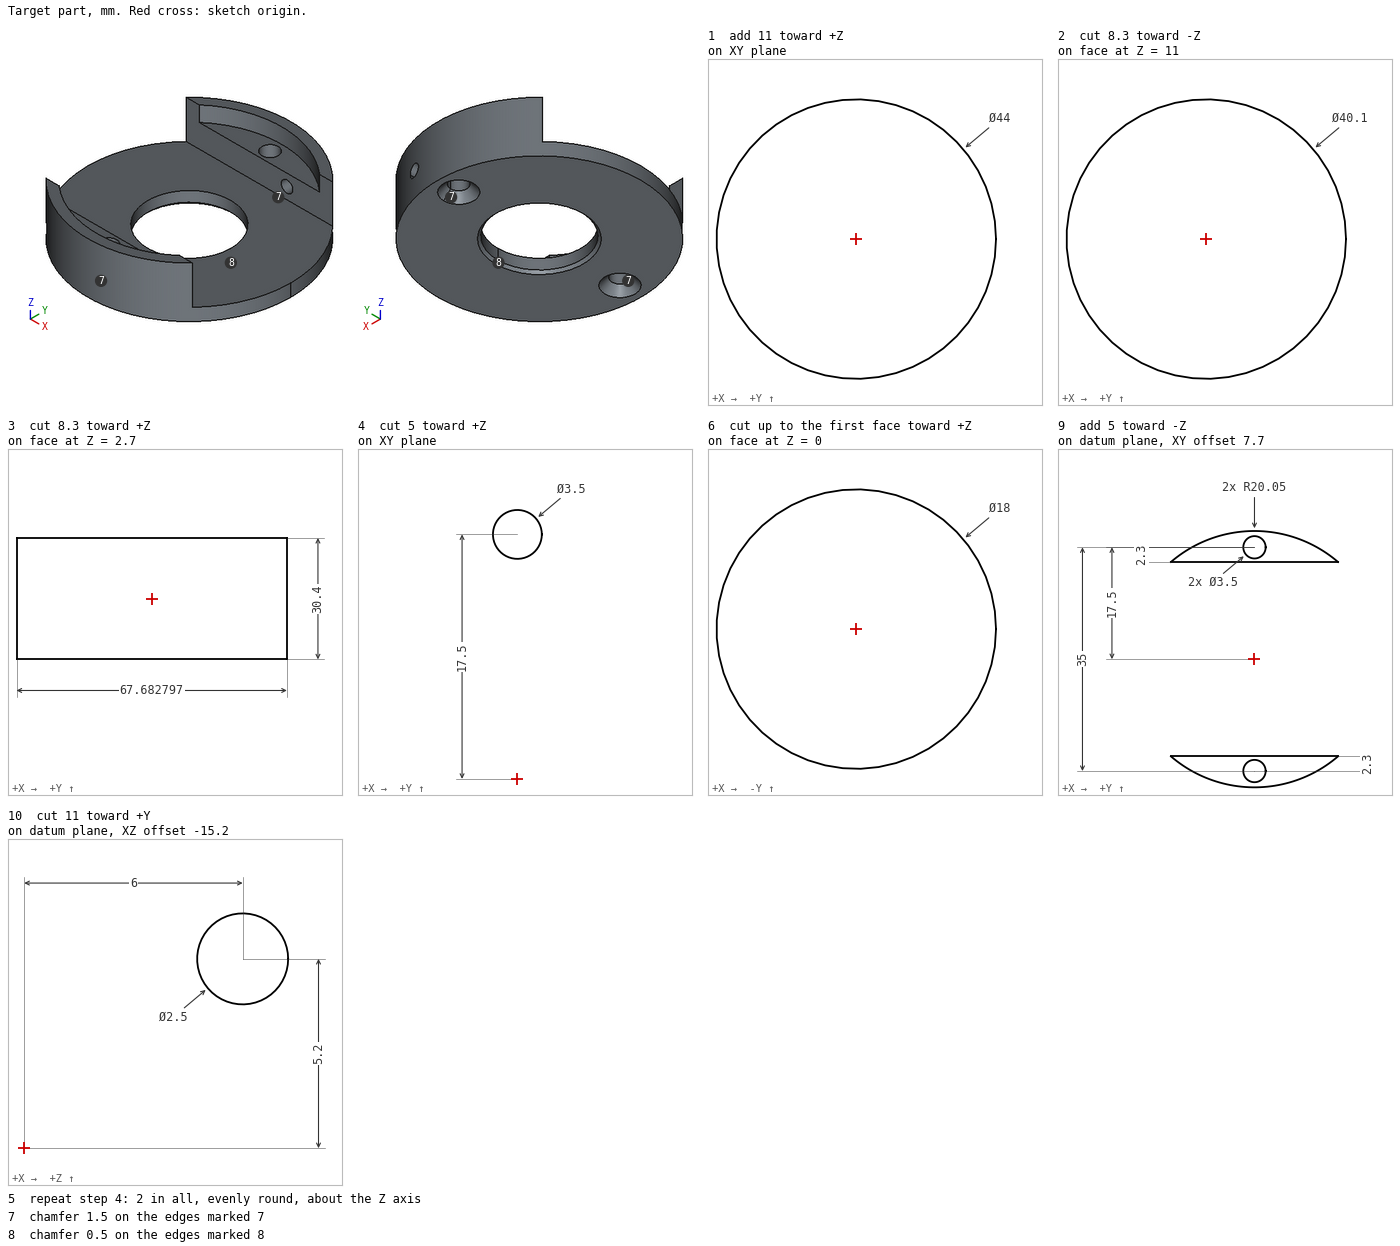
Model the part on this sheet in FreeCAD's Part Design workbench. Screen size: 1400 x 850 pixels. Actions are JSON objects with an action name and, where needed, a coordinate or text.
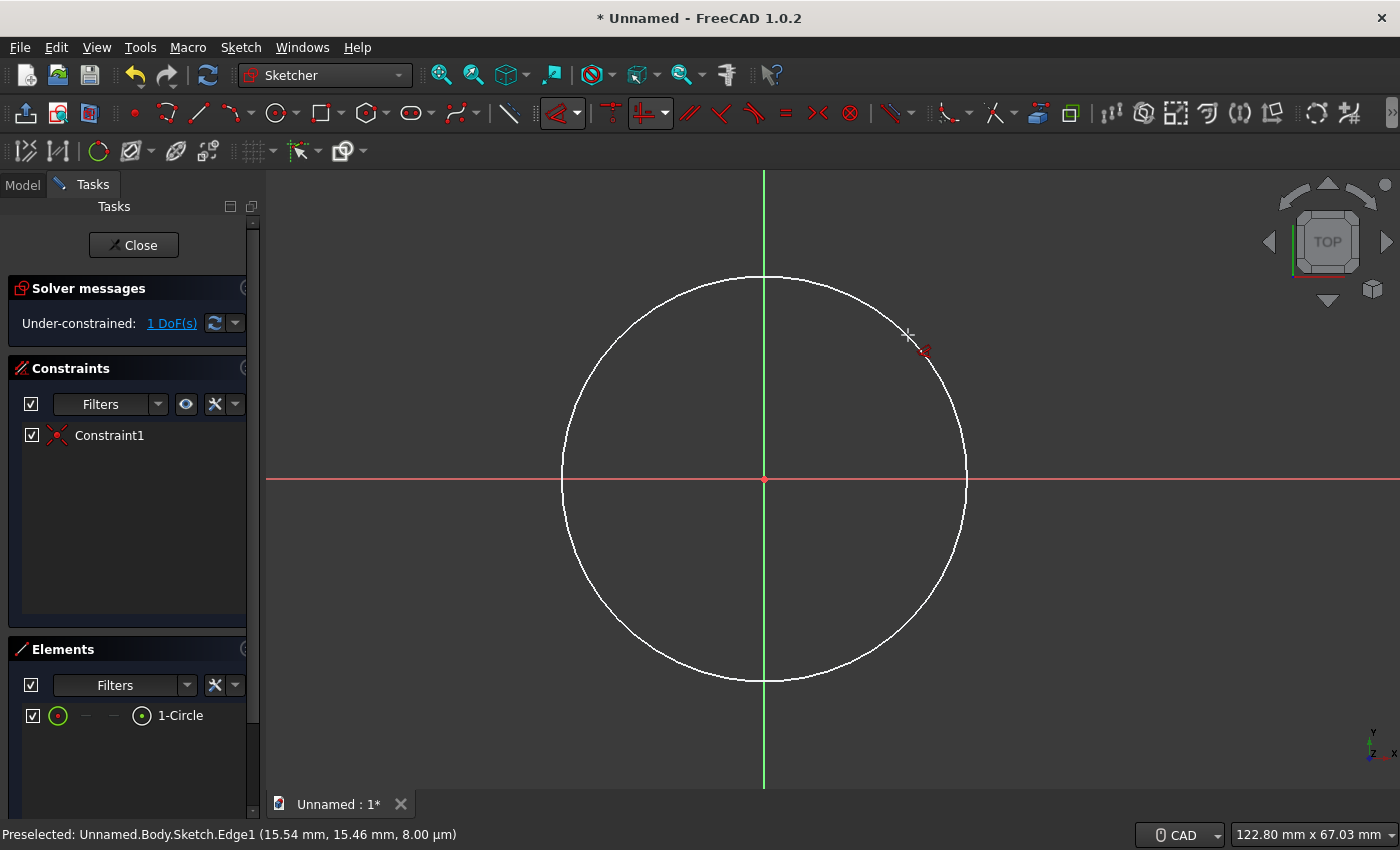
{"action": "left_click", "coordinate": [907, 335]}
{"action": "left_click", "coordinate": [930, 312]}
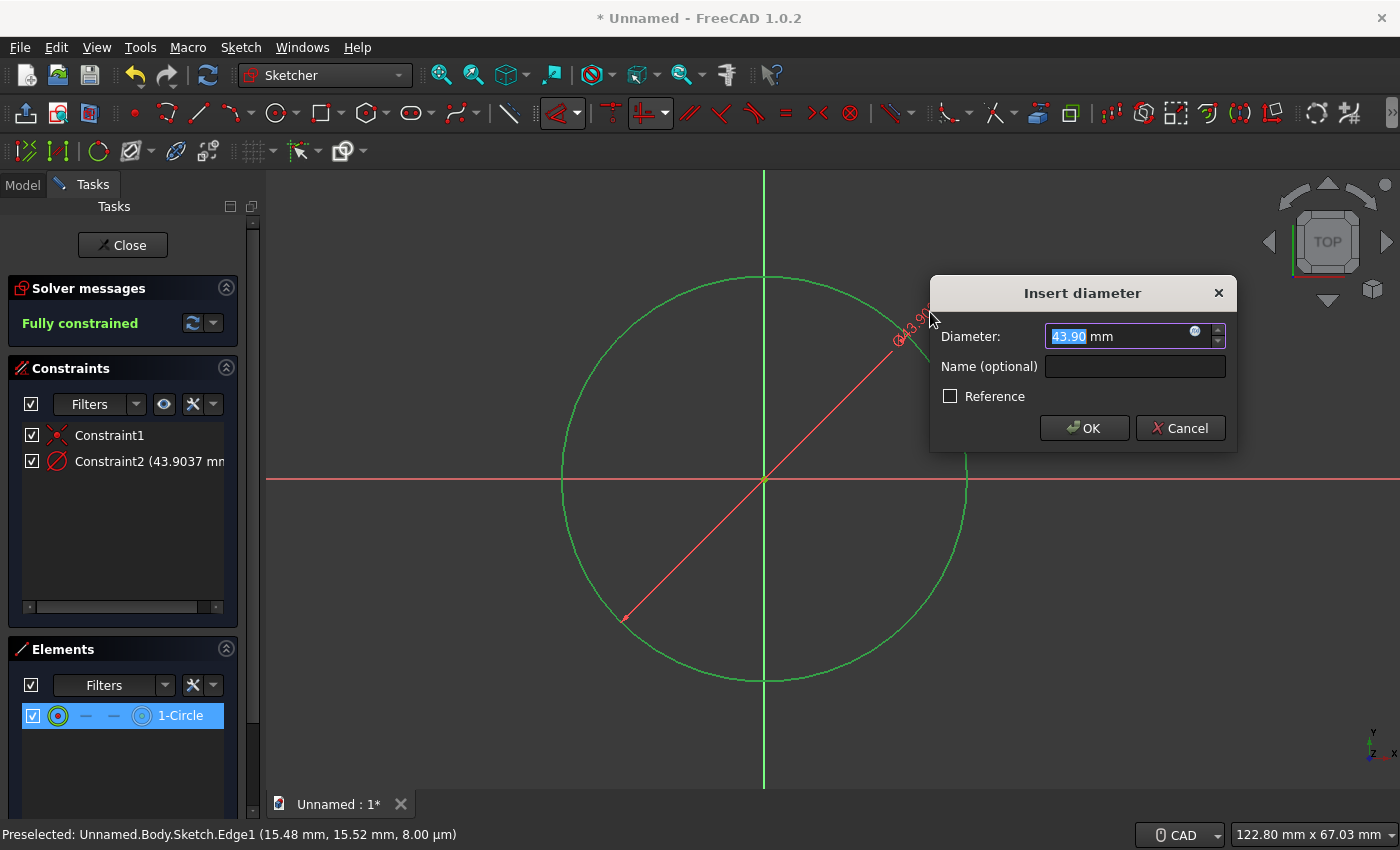
{"action": "type", "text": "44"}
{"action": "key", "text": "Return"}
{"action": "key", "text": "Escape"}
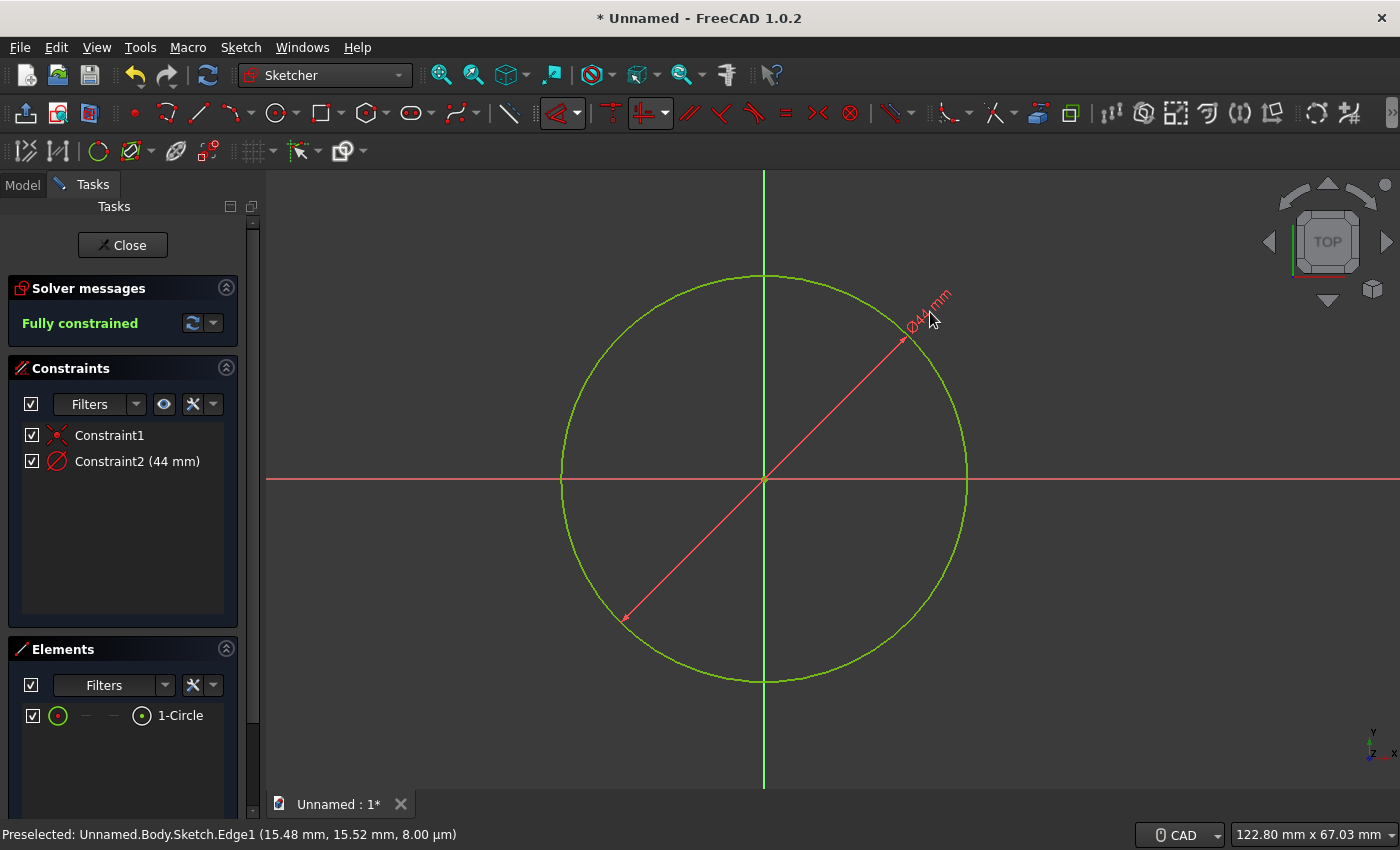
{"action": "left_click", "coordinate": [123, 245]}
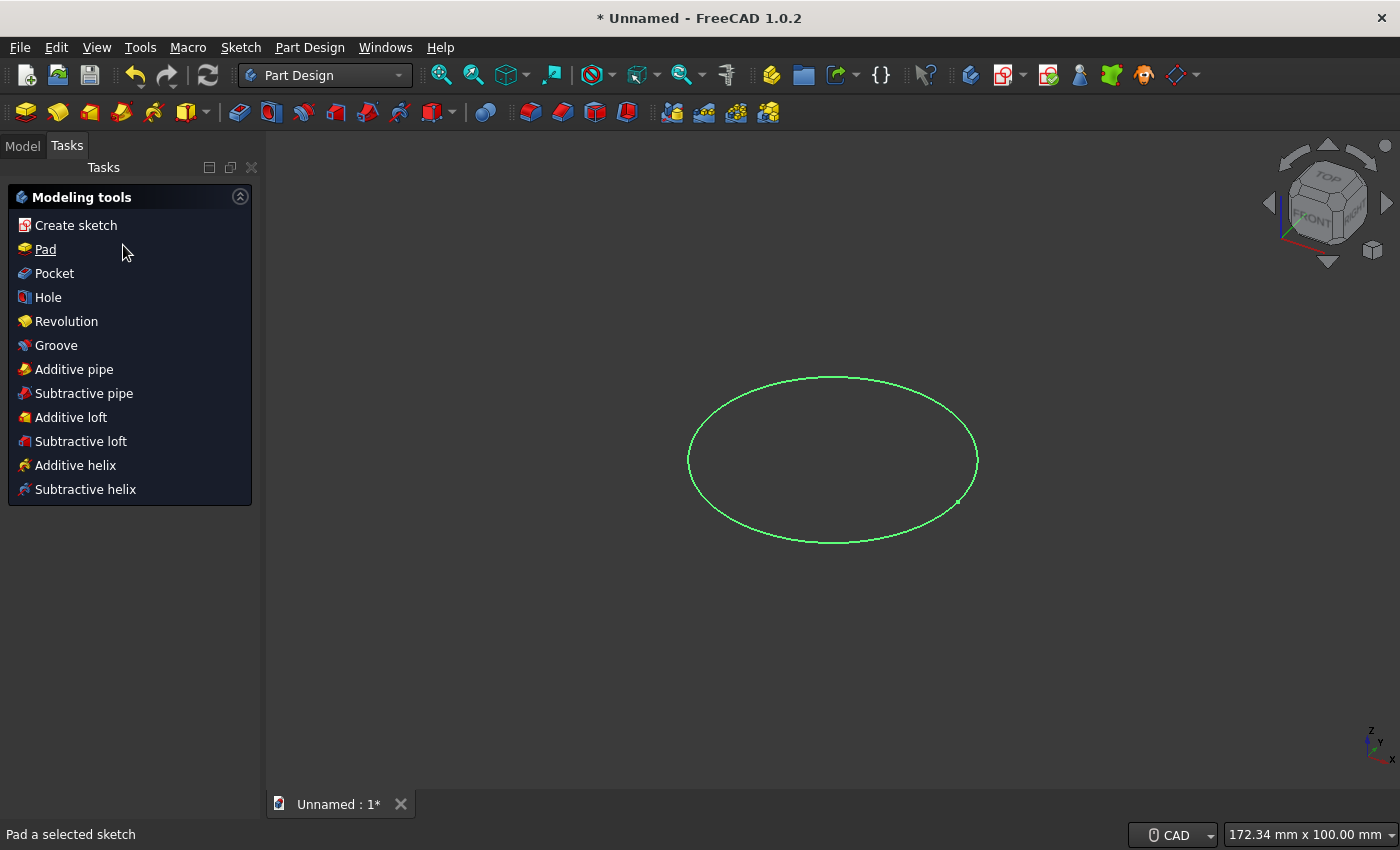
{"action": "left_click", "coordinate": [26, 112]}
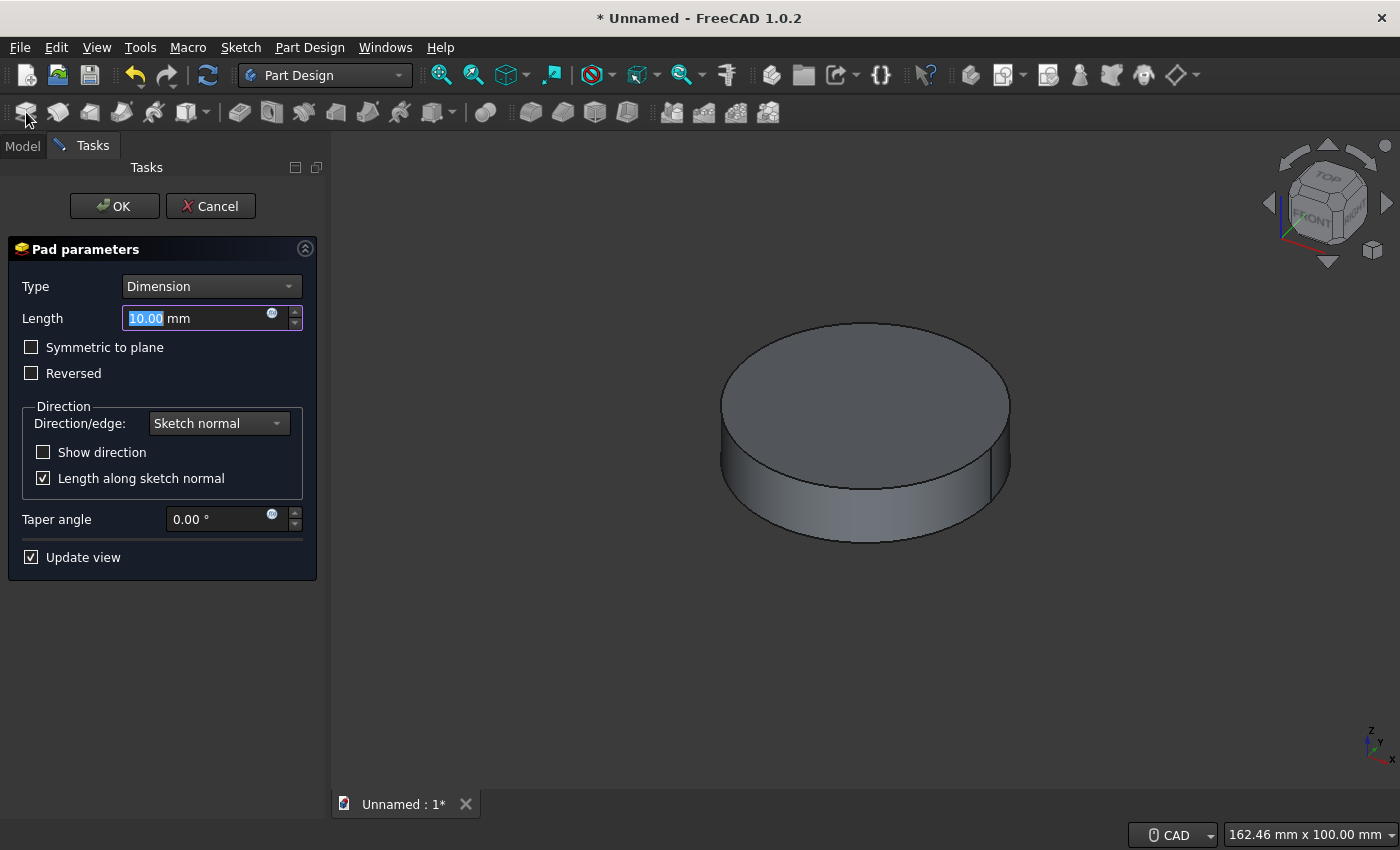
{"action": "type", "text": "11"}
{"action": "key", "text": "Tab"}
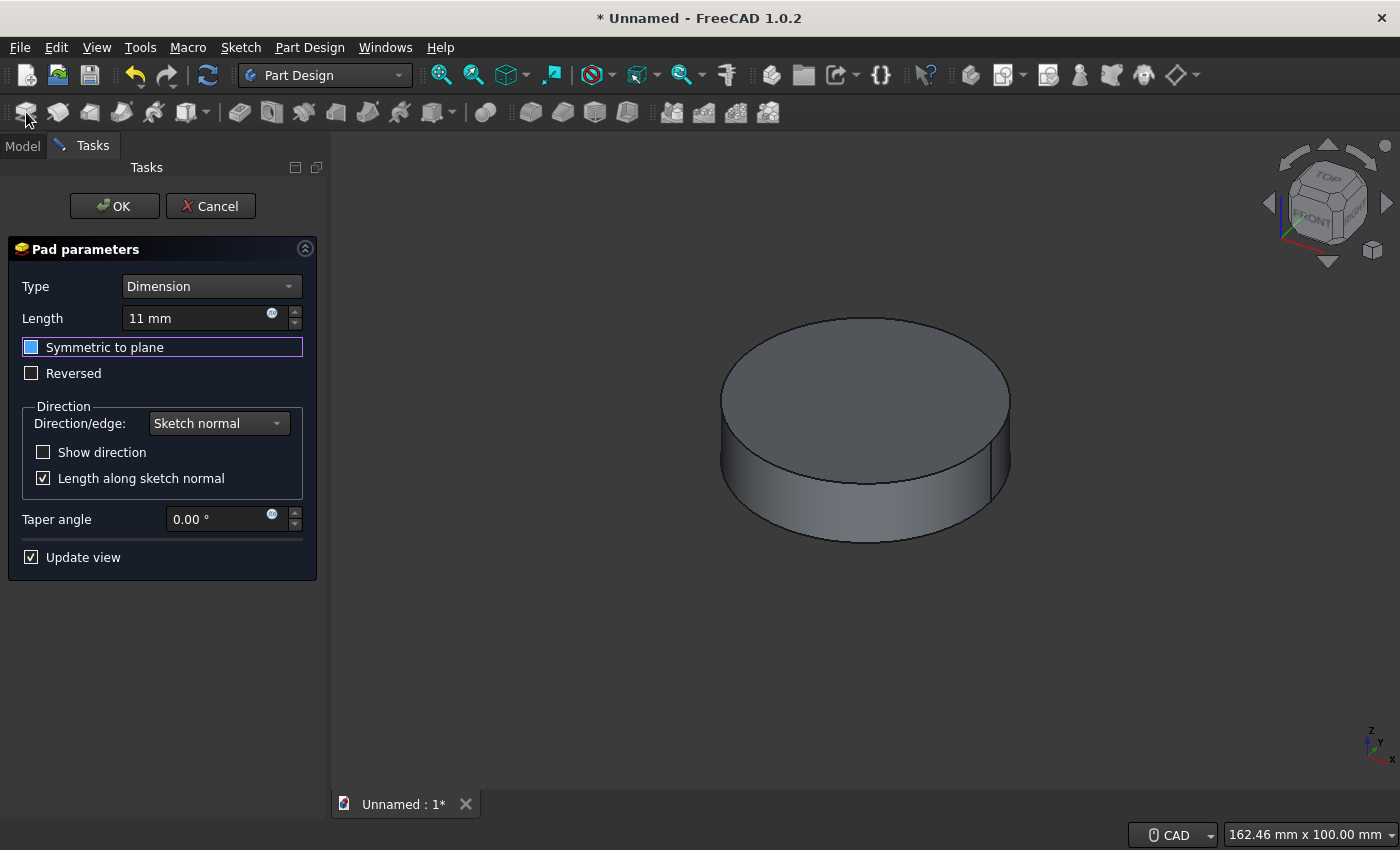
{"action": "left_click", "coordinate": [115, 206]}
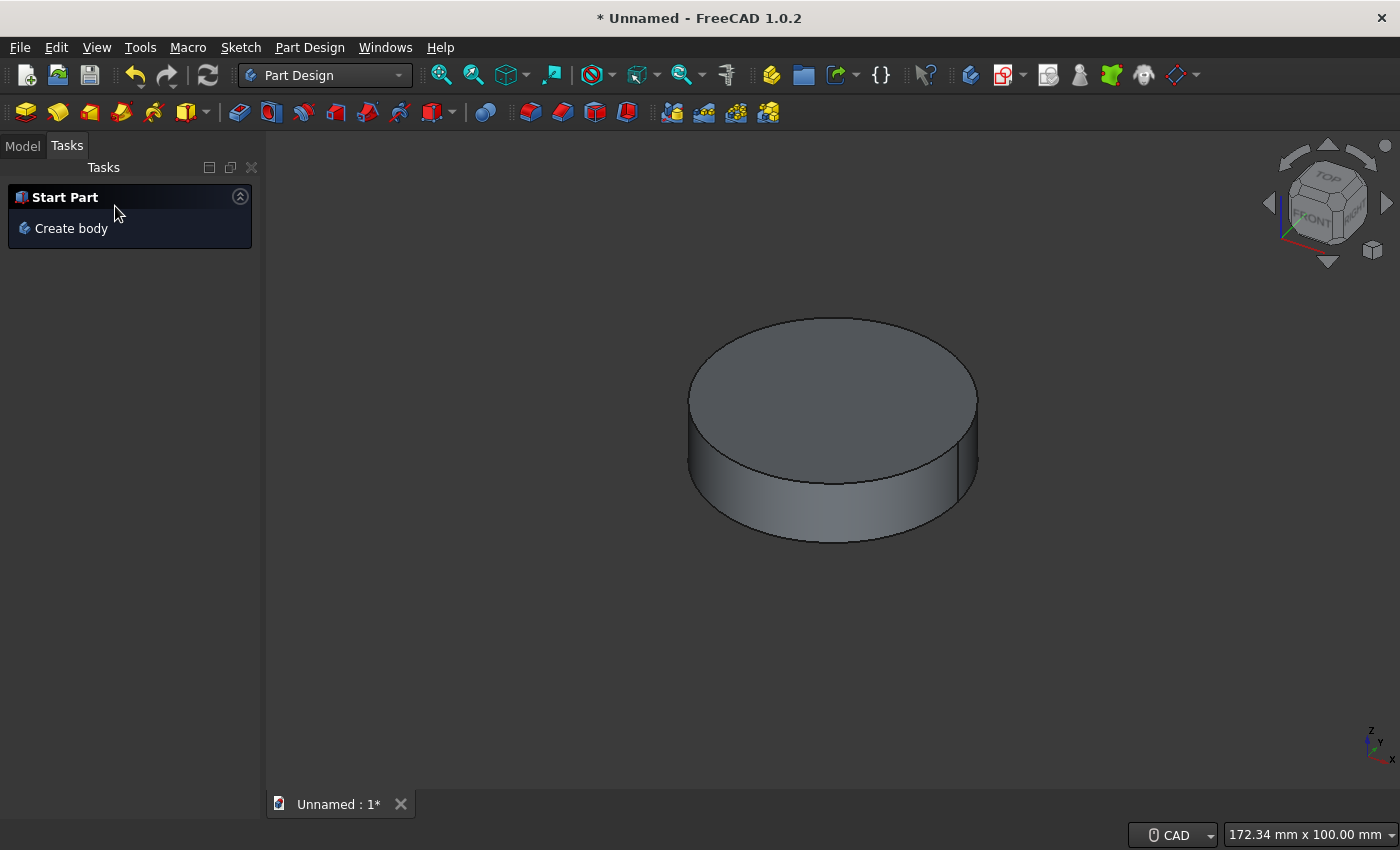
{"action": "key", "text": "v f"}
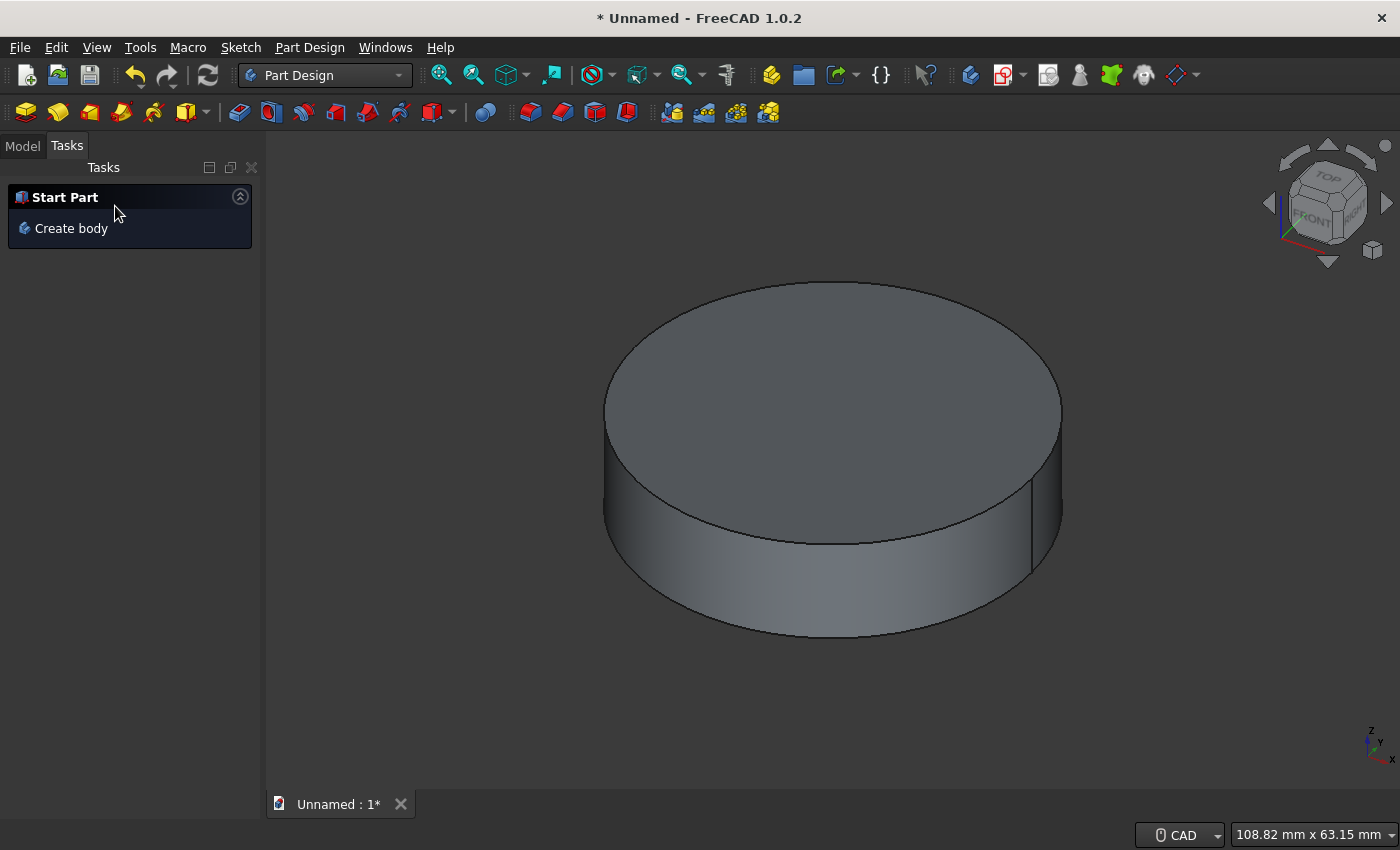
{"action": "left_click", "coordinate": [833, 412]}